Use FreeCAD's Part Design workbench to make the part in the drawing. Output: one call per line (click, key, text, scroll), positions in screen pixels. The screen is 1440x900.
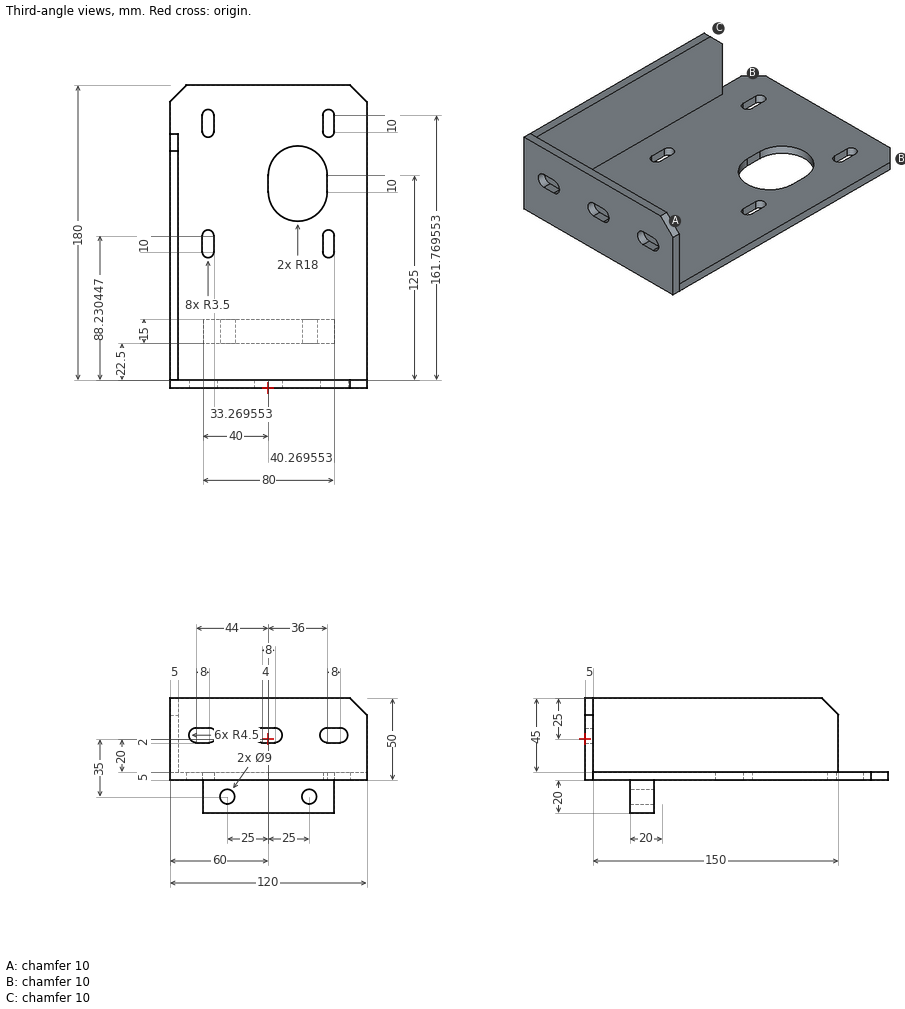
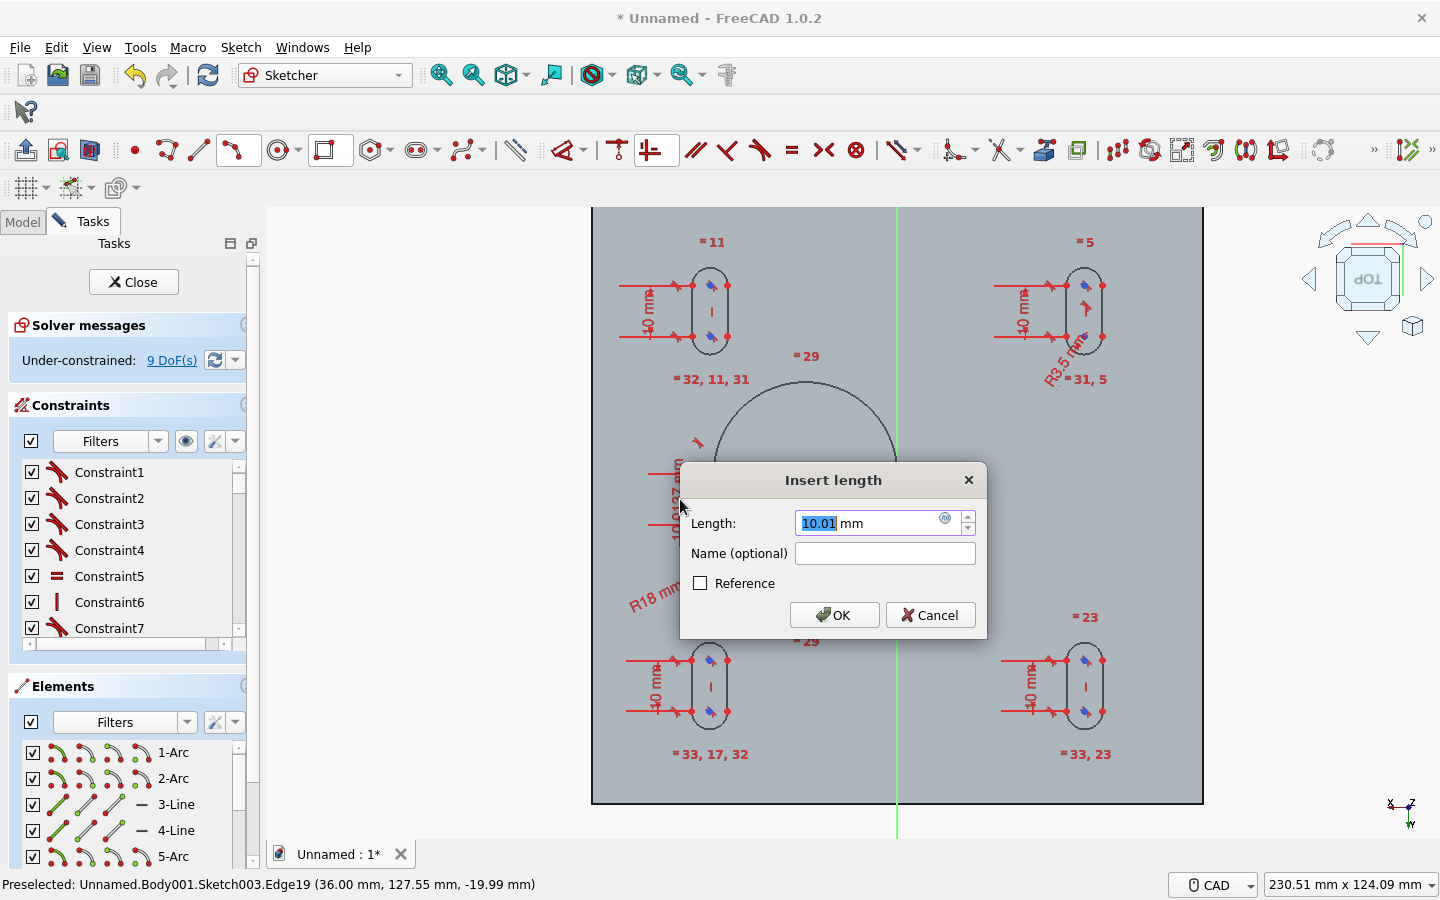
text(10)
key(Return)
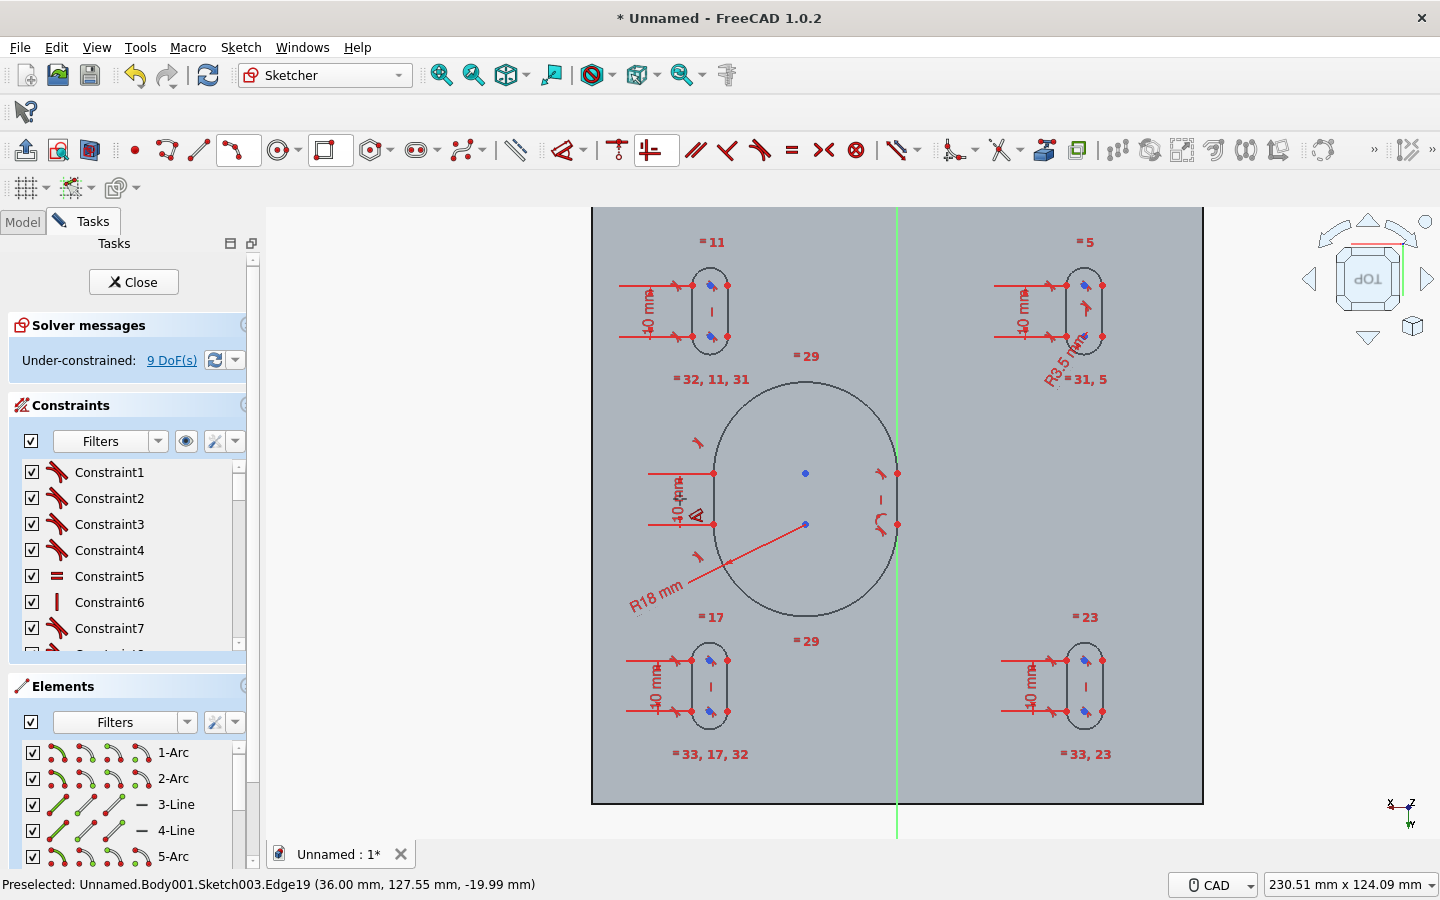
click(714, 525)
click(680, 380)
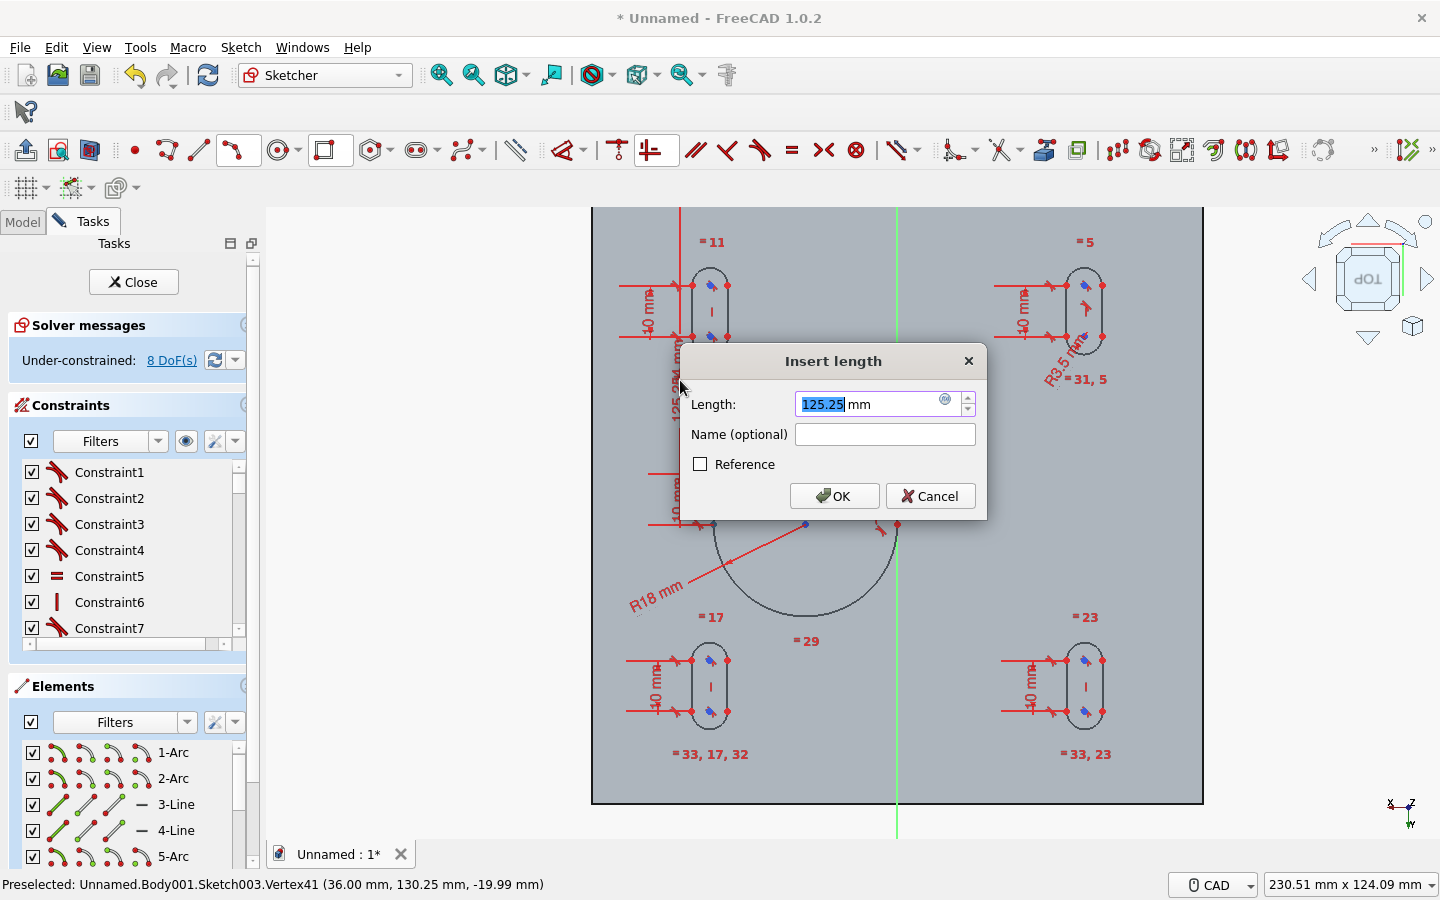
text(125)
key(Return)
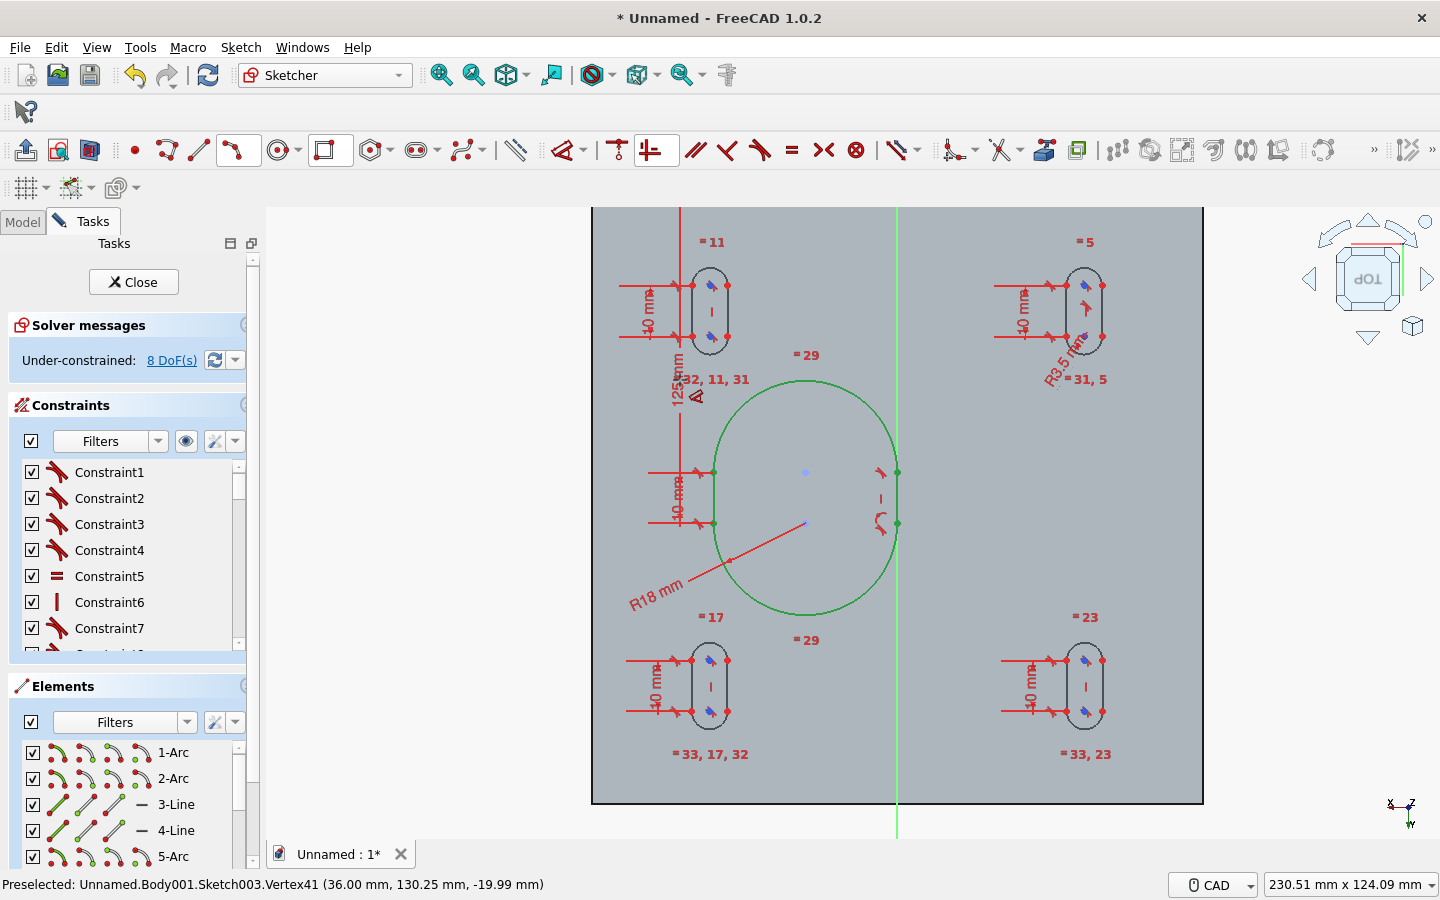
click(1066, 337)
click(982, 371)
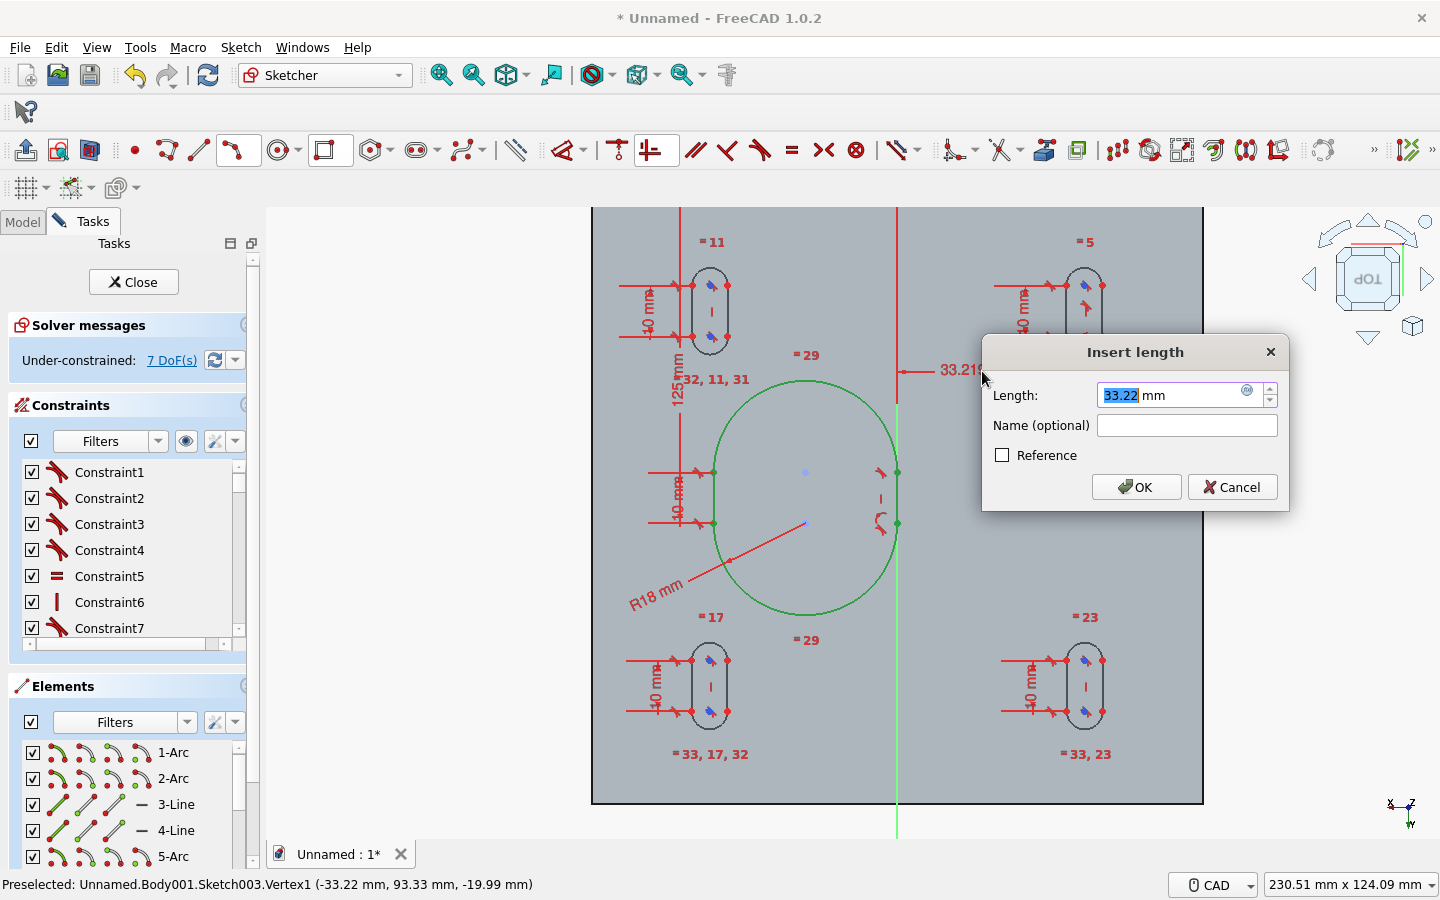
text(33.269553)
key(Return)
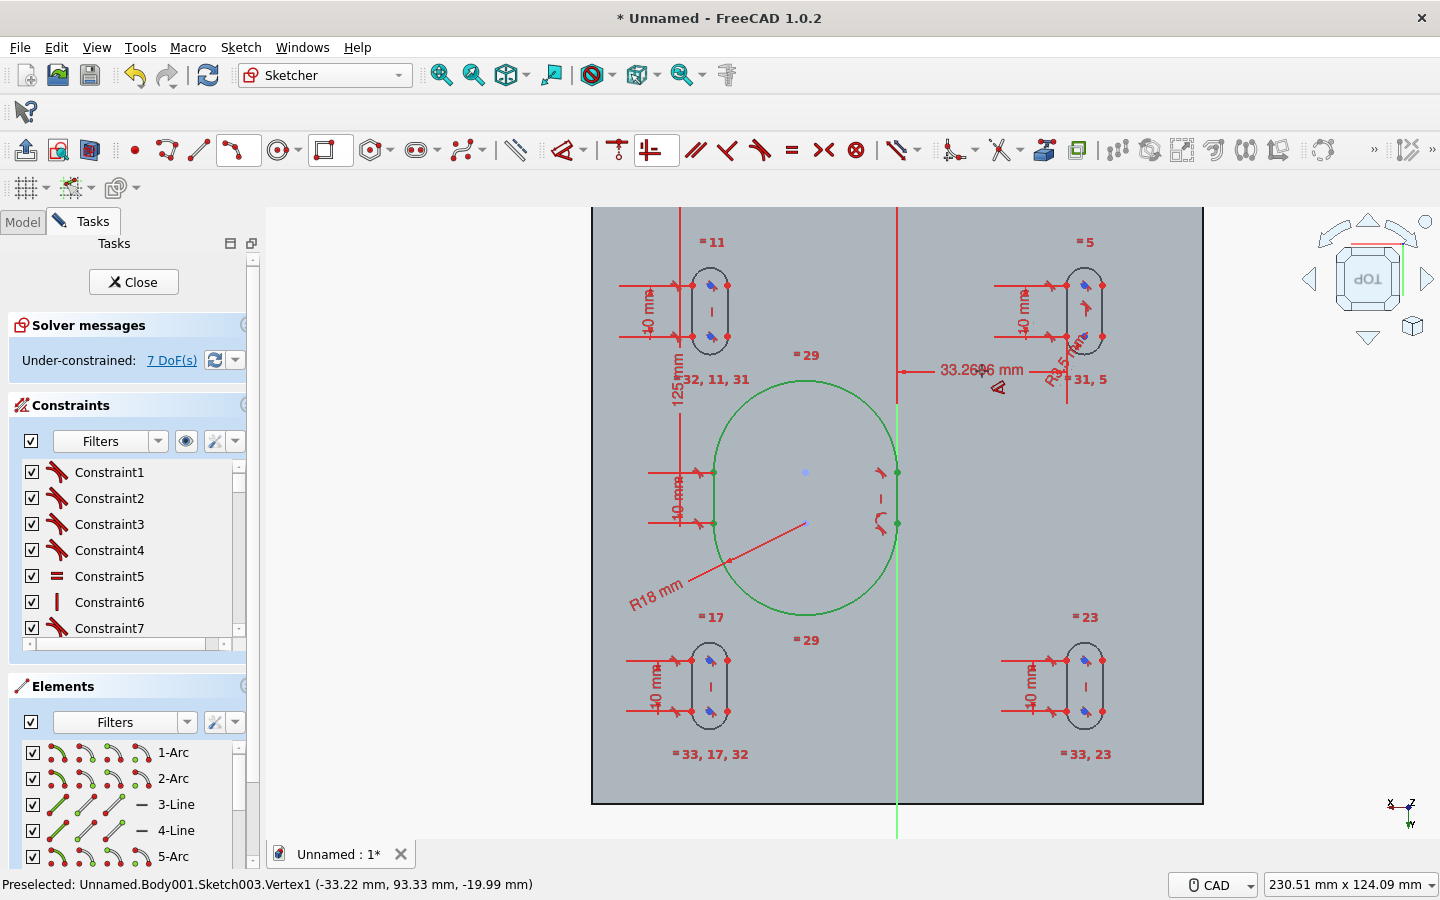
click(1067, 337)
click(1101, 250)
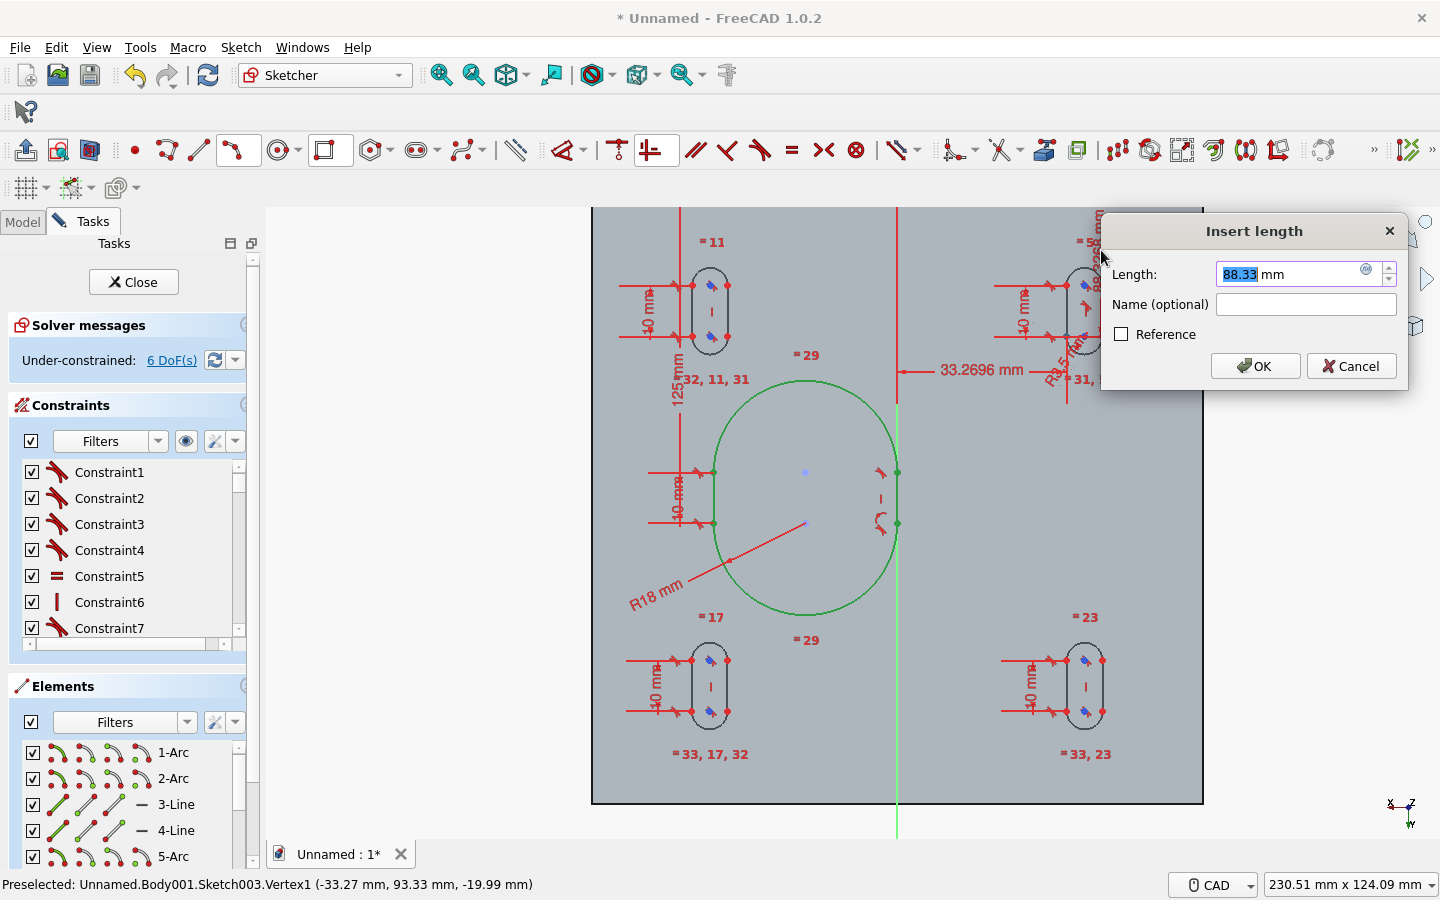
text(88.230447)
key(Return)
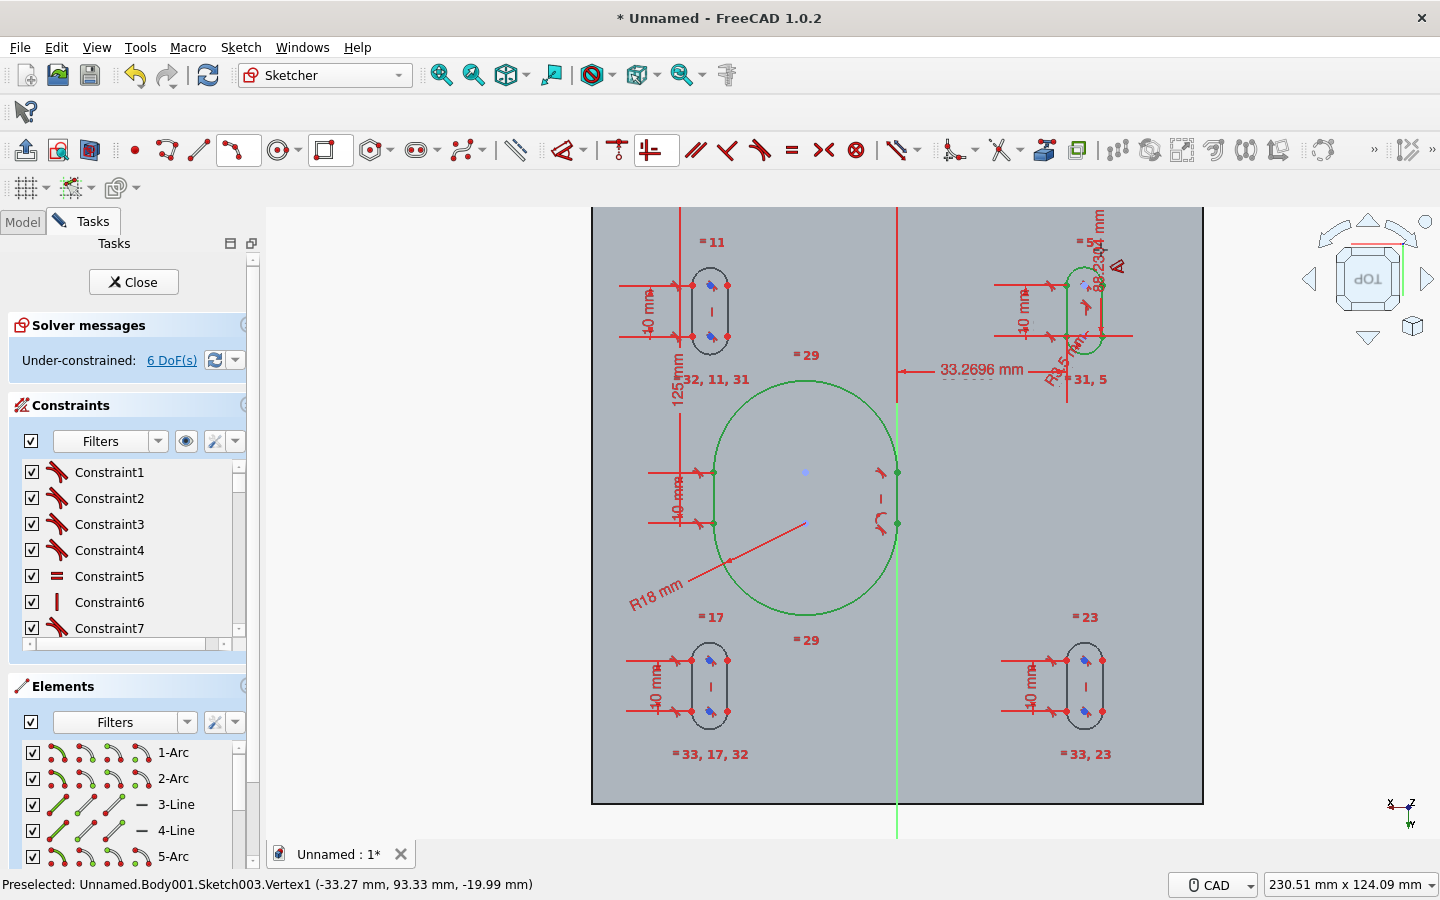
click(692, 337)
click(842, 371)